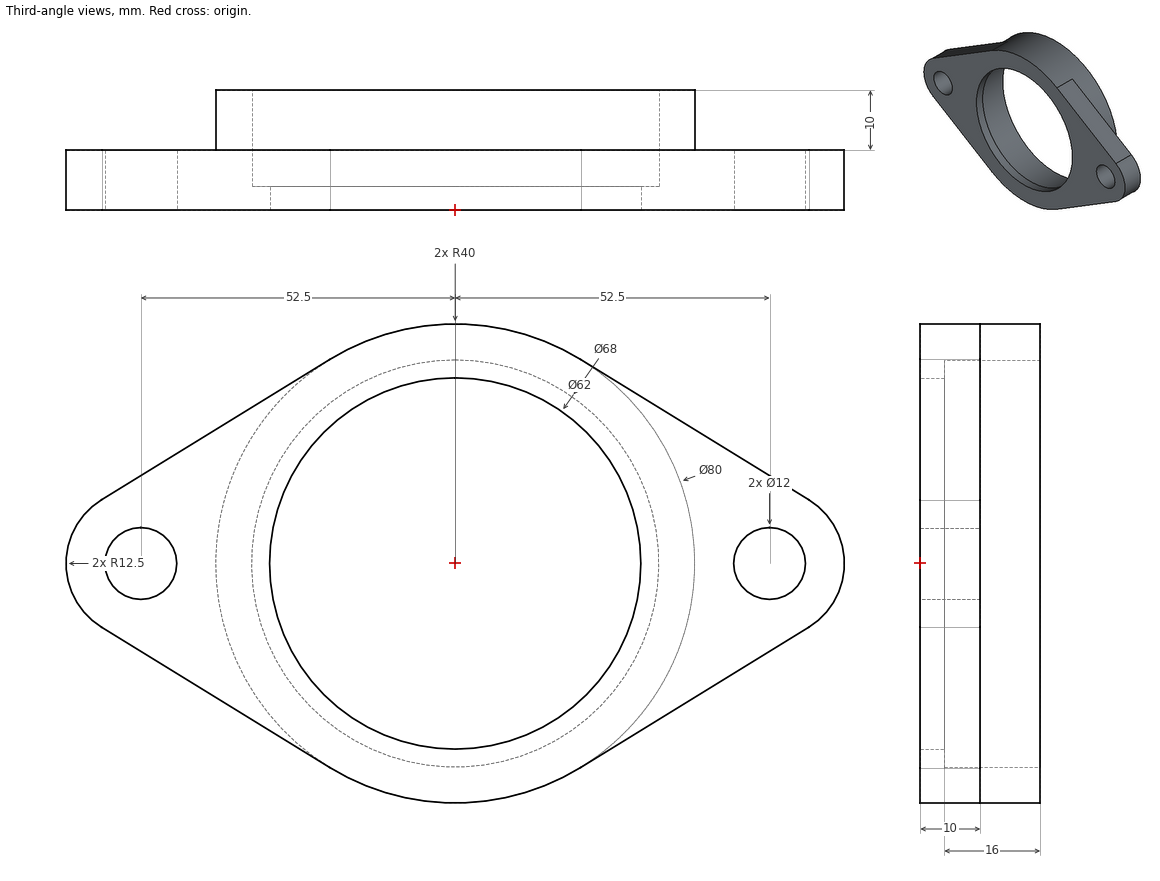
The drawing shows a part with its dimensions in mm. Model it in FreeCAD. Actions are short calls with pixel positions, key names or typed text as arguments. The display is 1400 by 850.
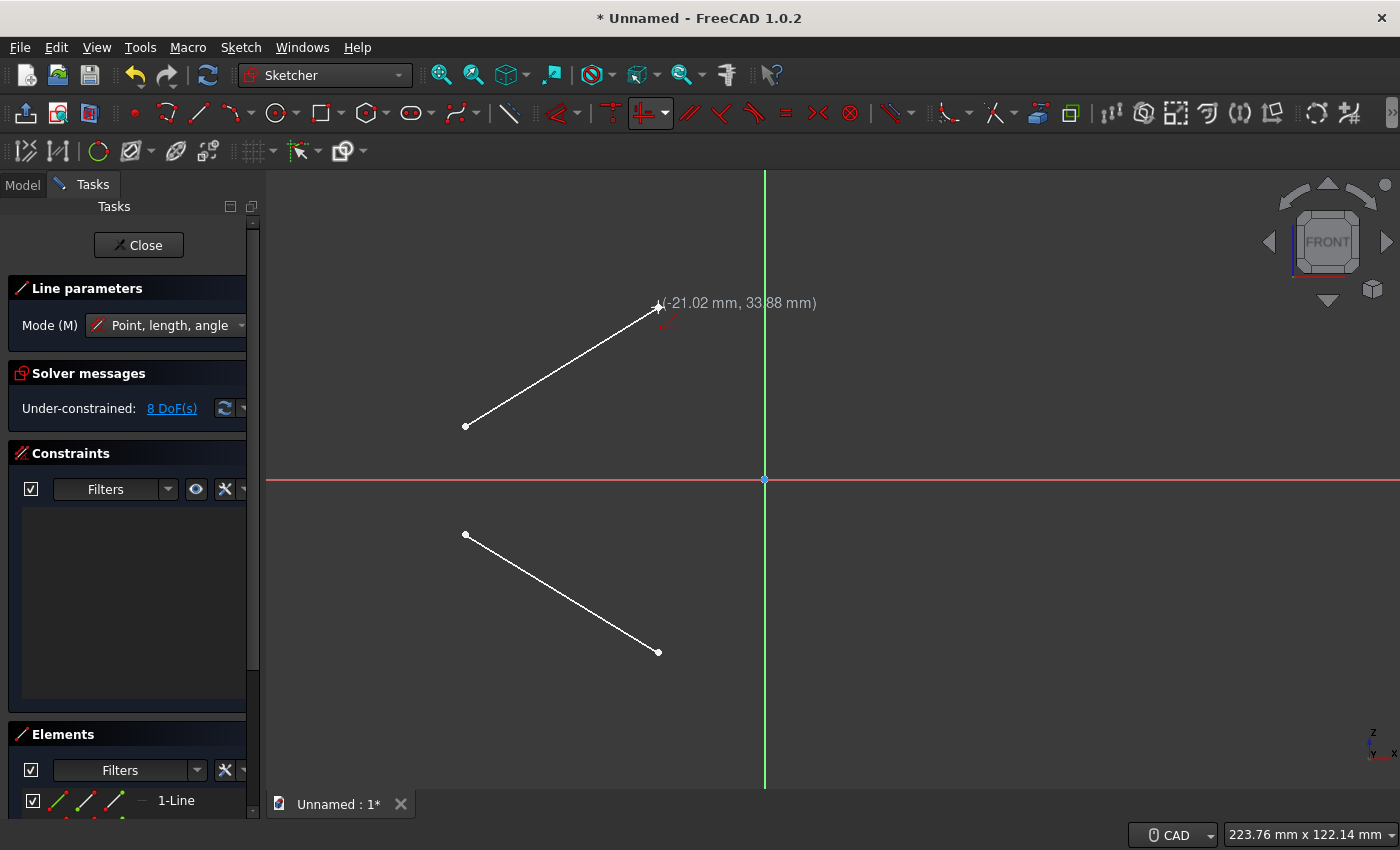
click(871, 307)
click(1064, 426)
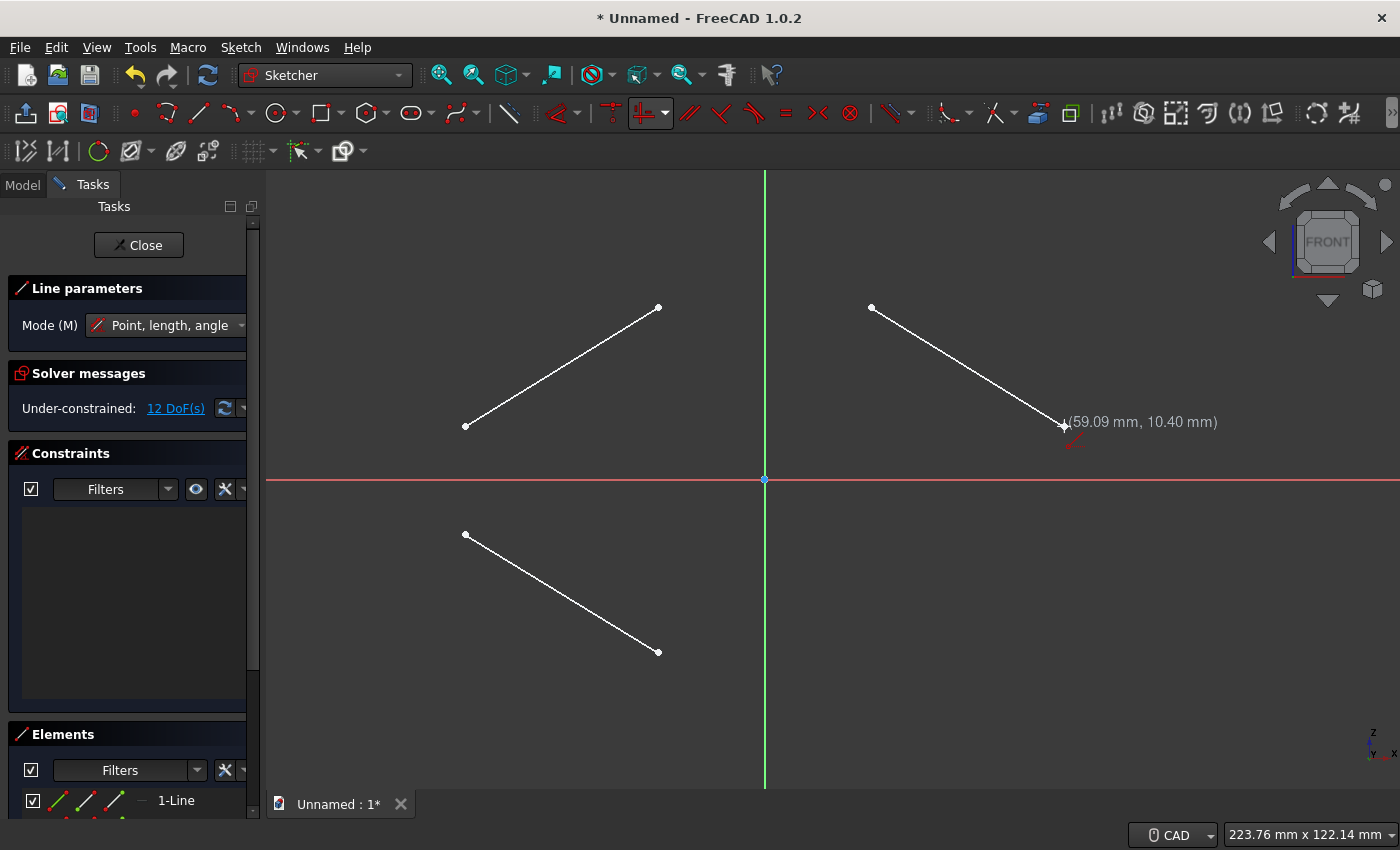
click(1064, 534)
click(871, 652)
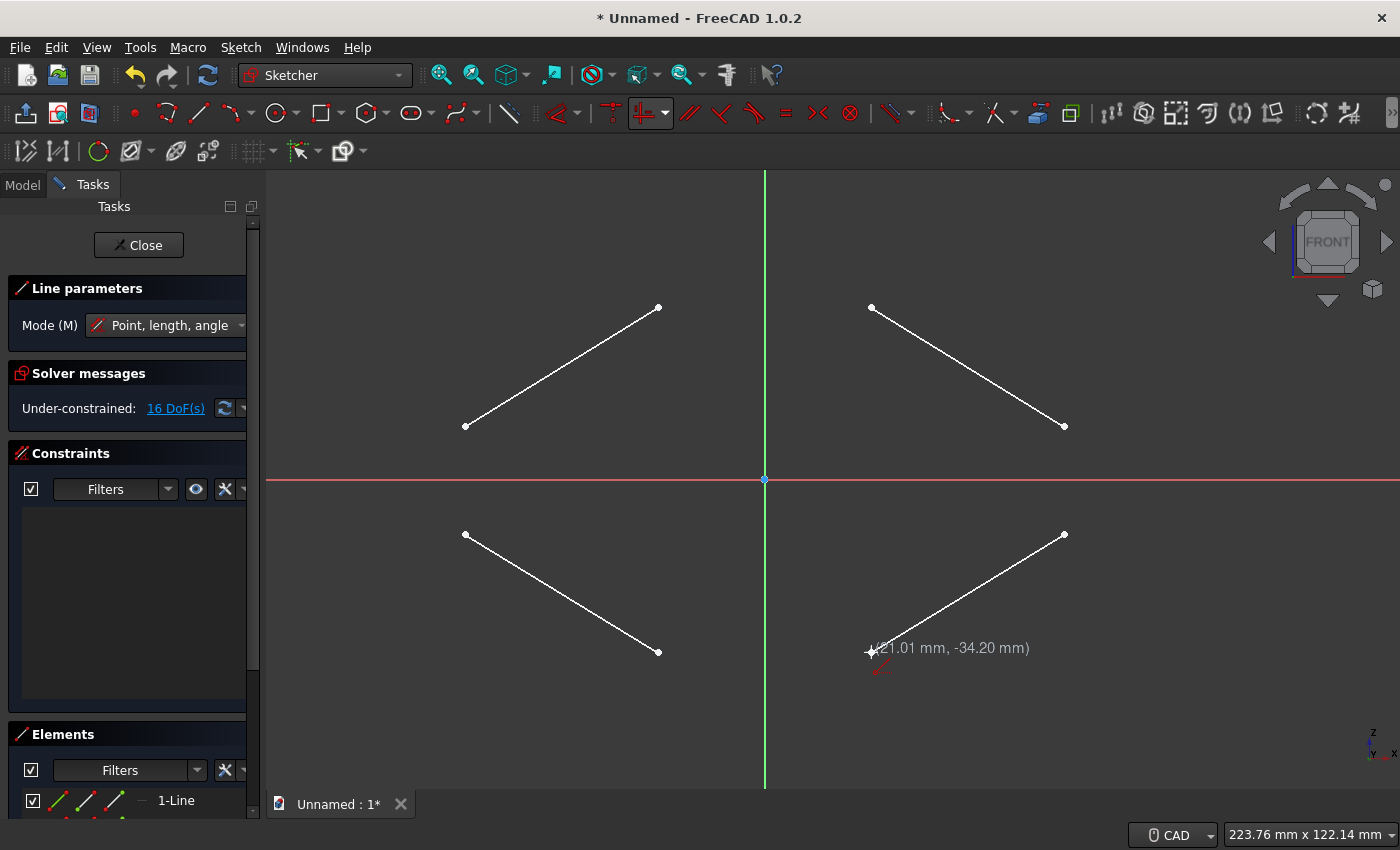
click(232, 114)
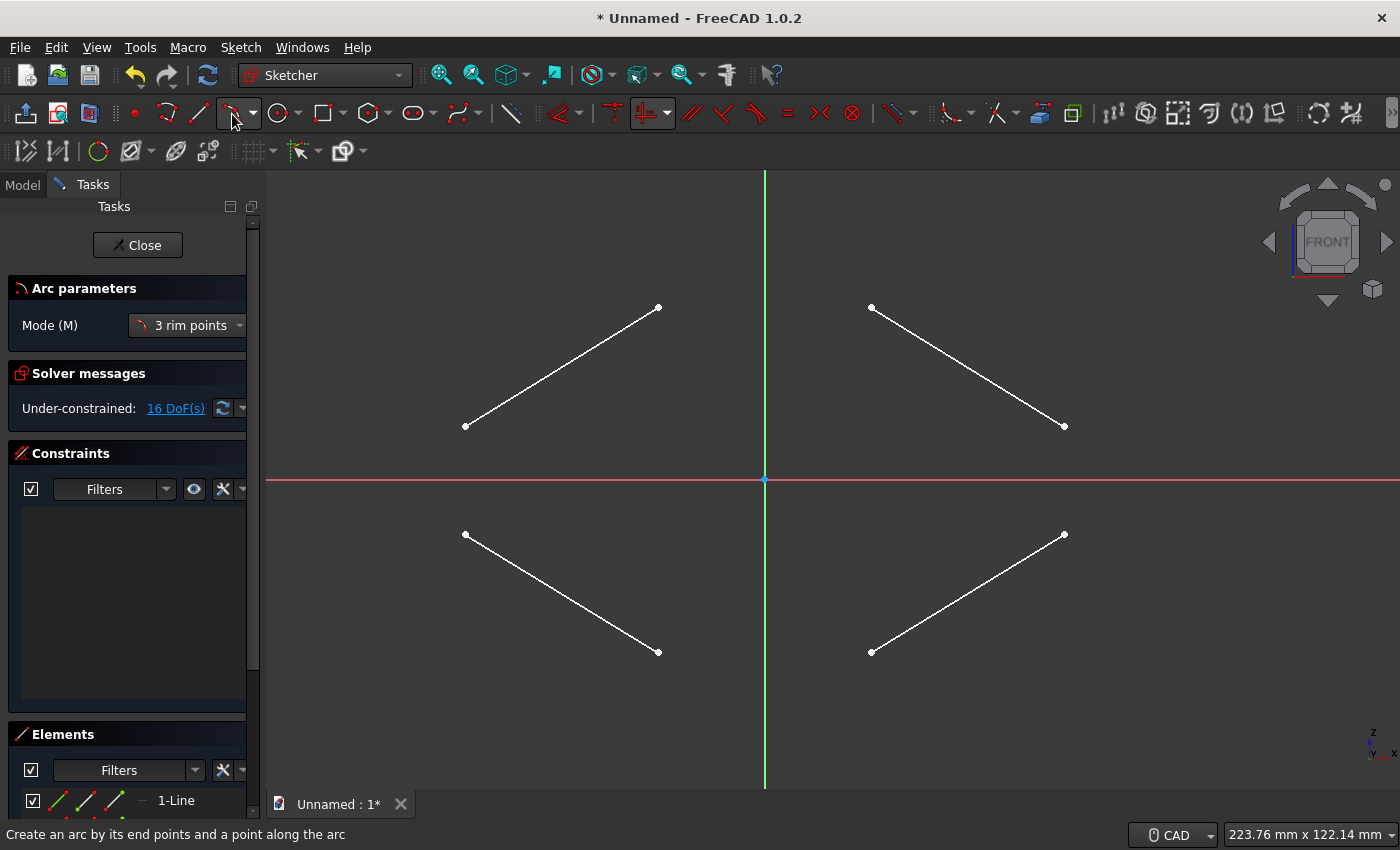
click(465, 535)
click(465, 427)
click(440, 455)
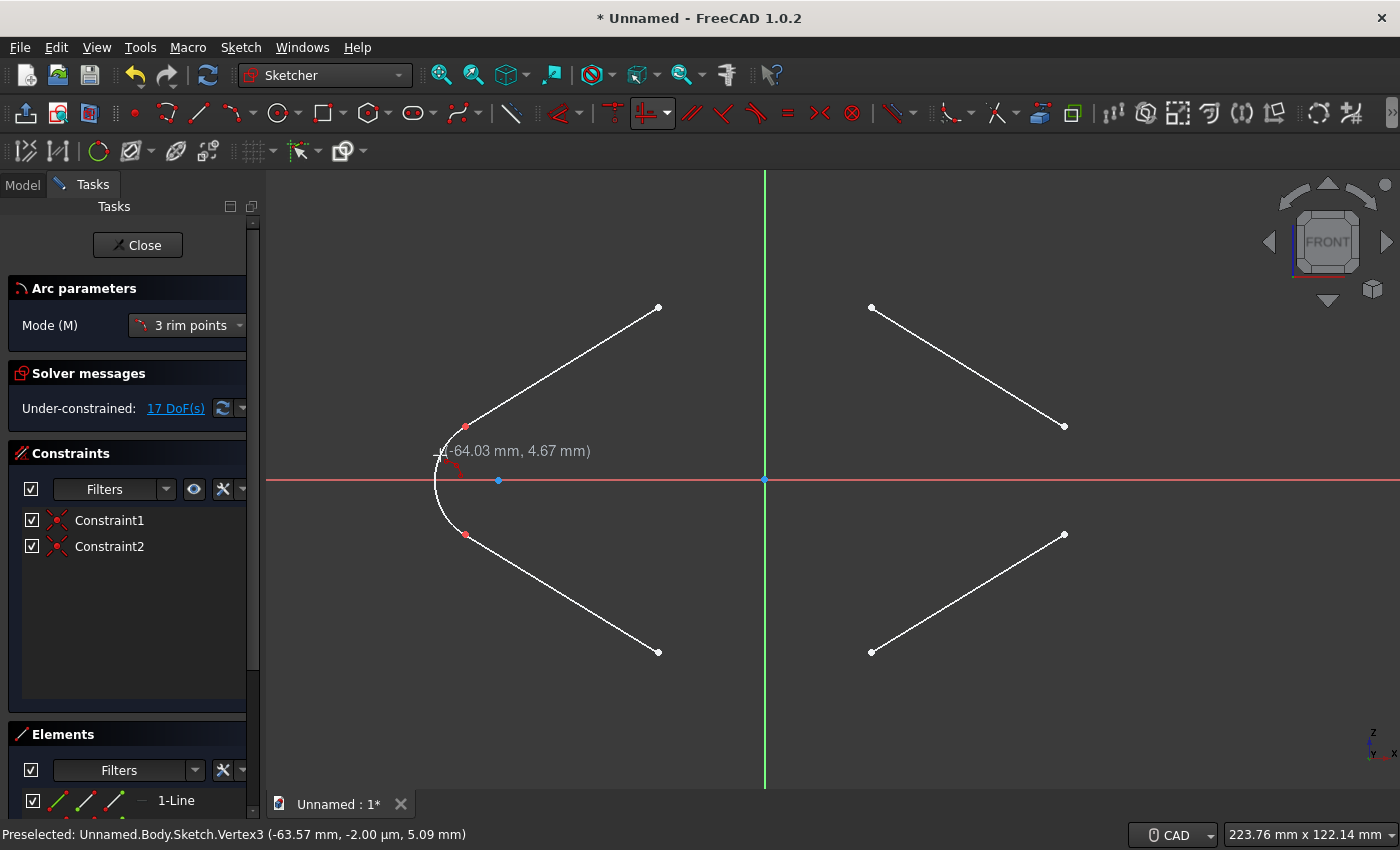
click(658, 308)
click(871, 308)
click(787, 278)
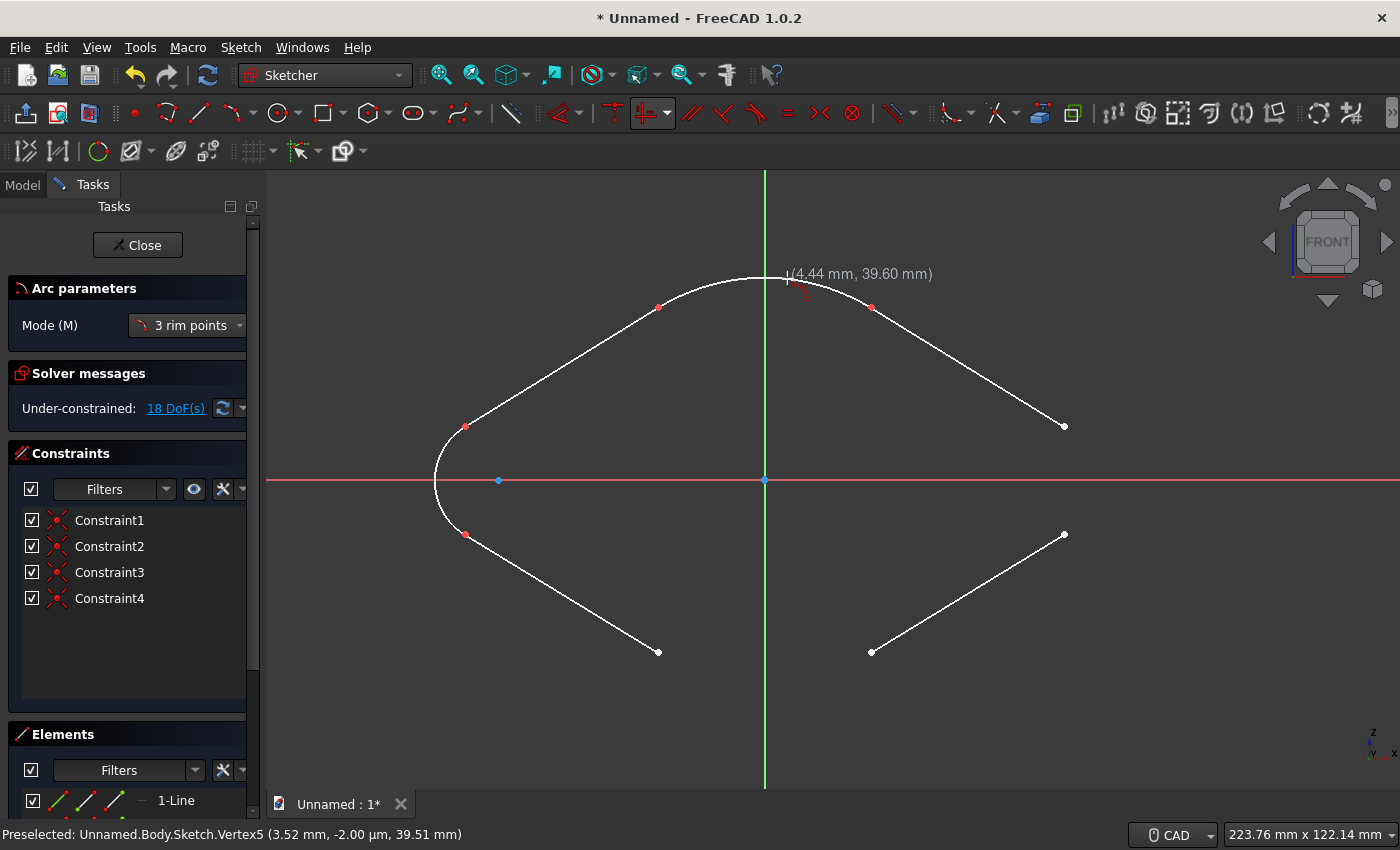
click(1064, 427)
click(1064, 535)
click(1089, 505)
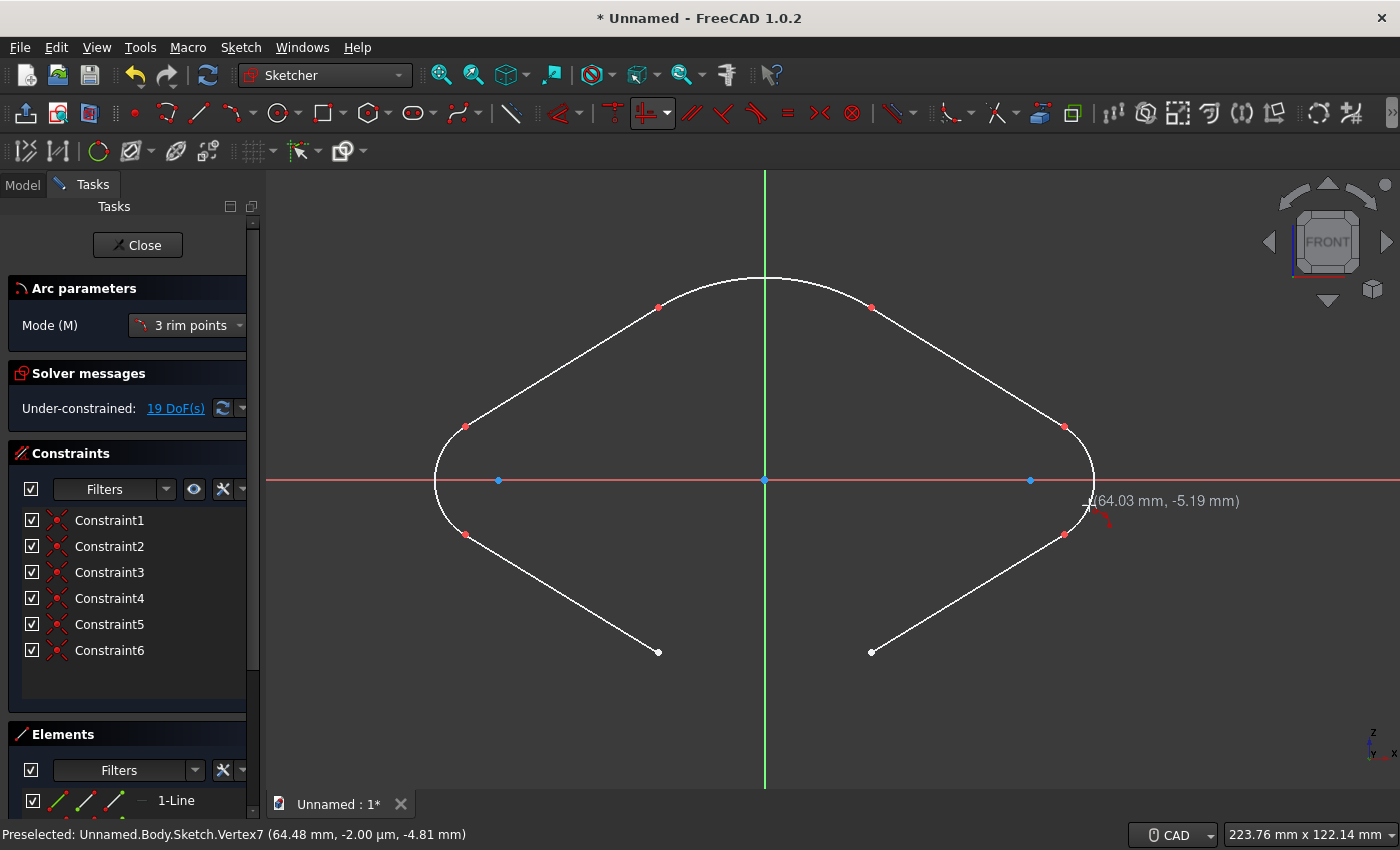
click(871, 653)
click(658, 653)
click(742, 681)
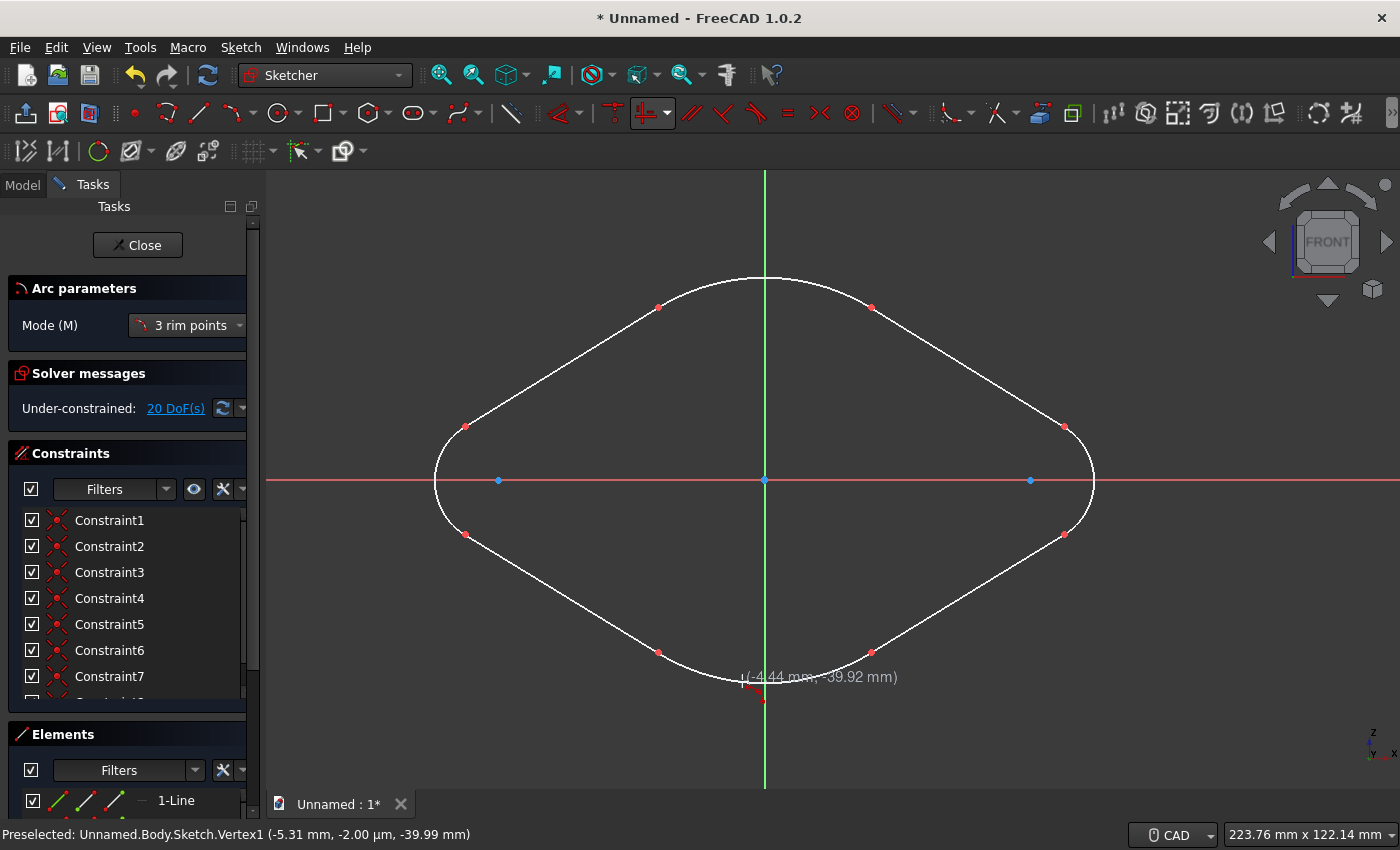
click(278, 114)